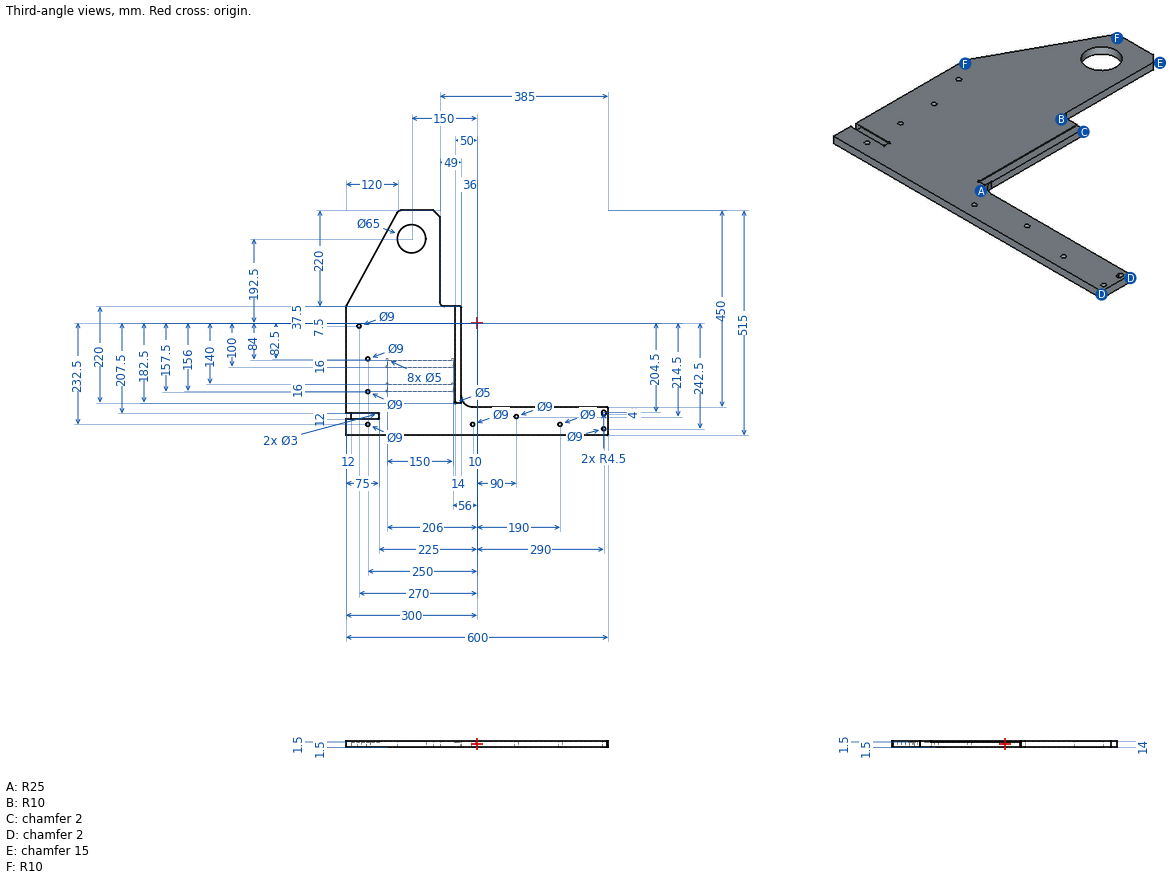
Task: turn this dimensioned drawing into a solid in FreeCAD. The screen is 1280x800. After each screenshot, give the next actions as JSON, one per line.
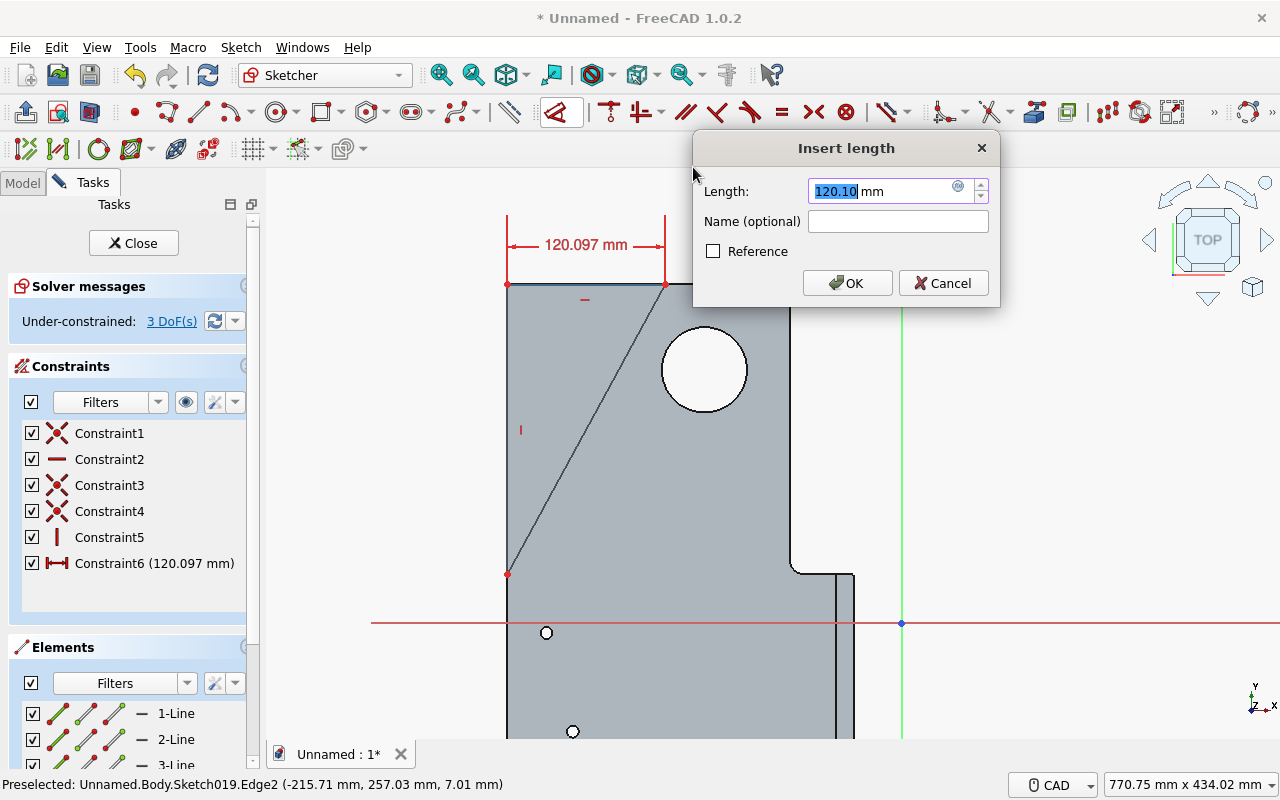
{"action": "type", "text": "120"}
{"action": "key", "text": "Return"}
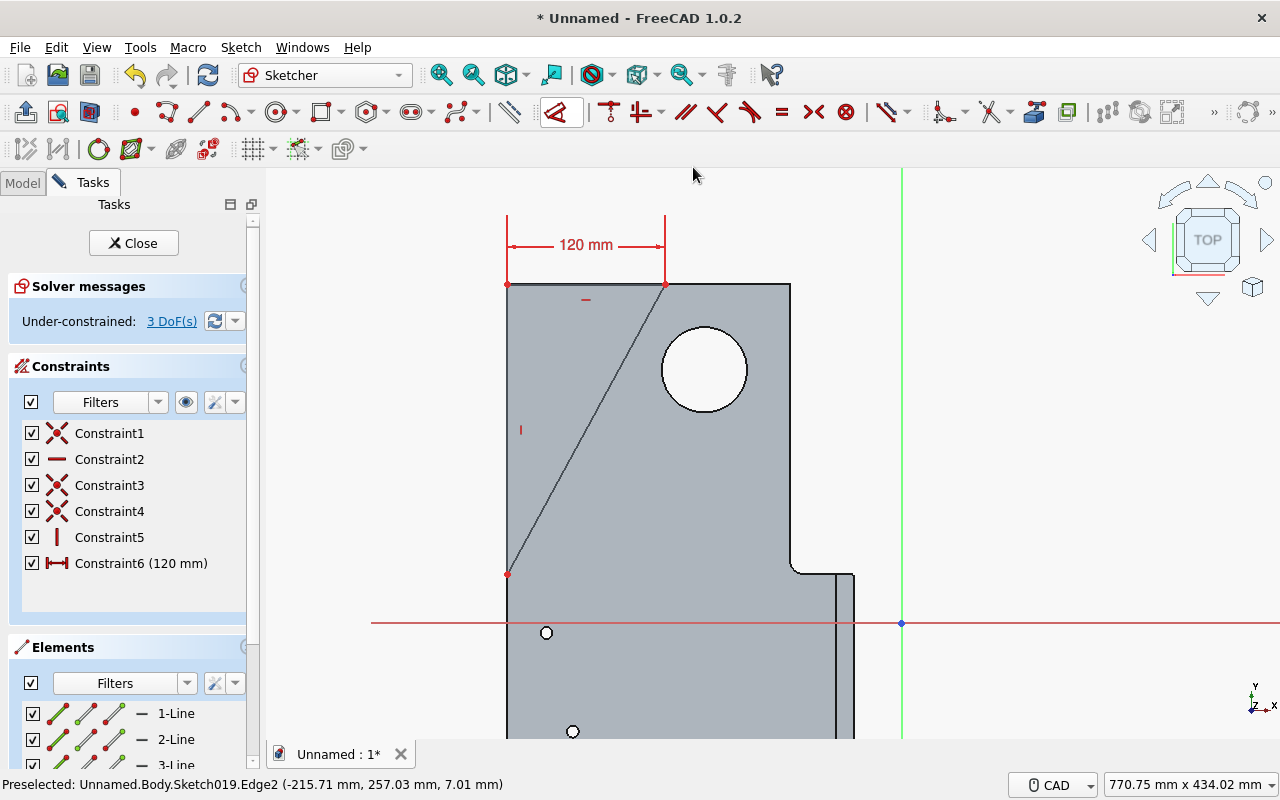
{"action": "left_click", "coordinate": [507, 372]}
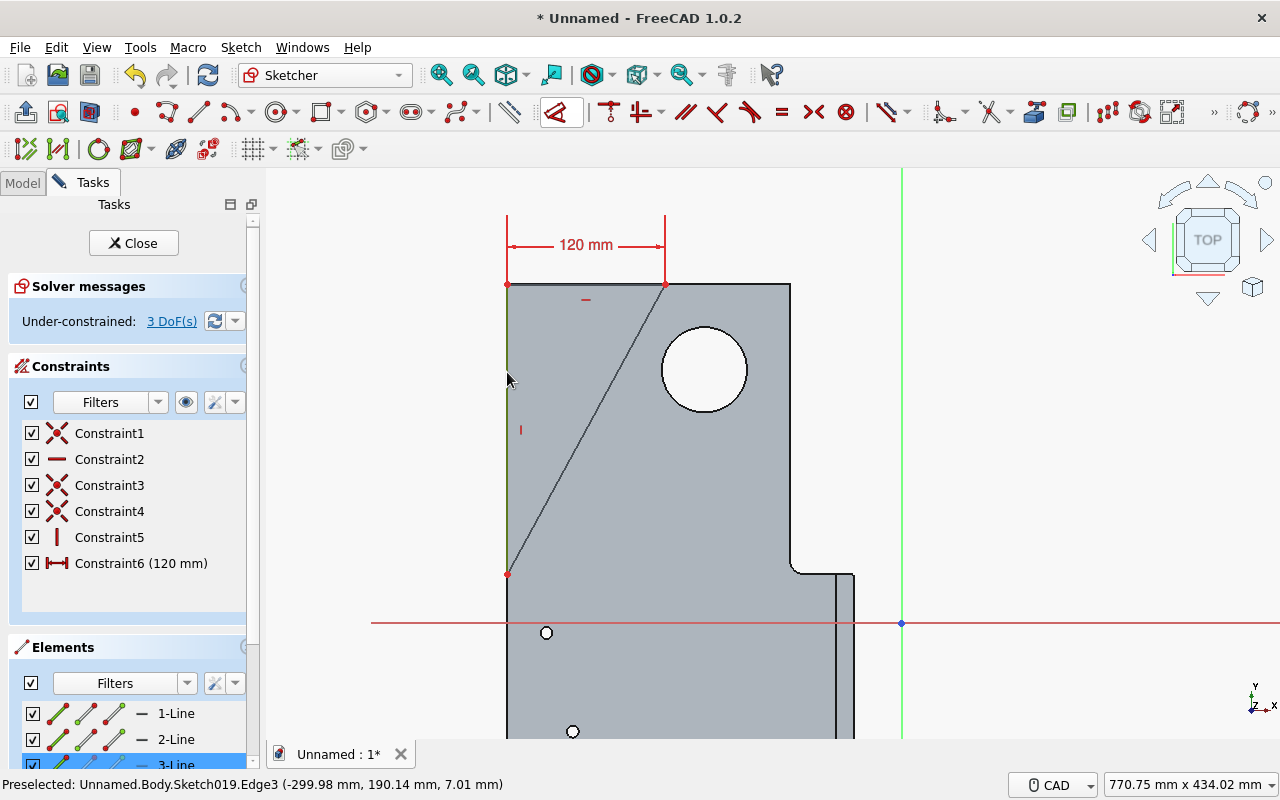
{"action": "left_click", "coordinate": [578, 112]}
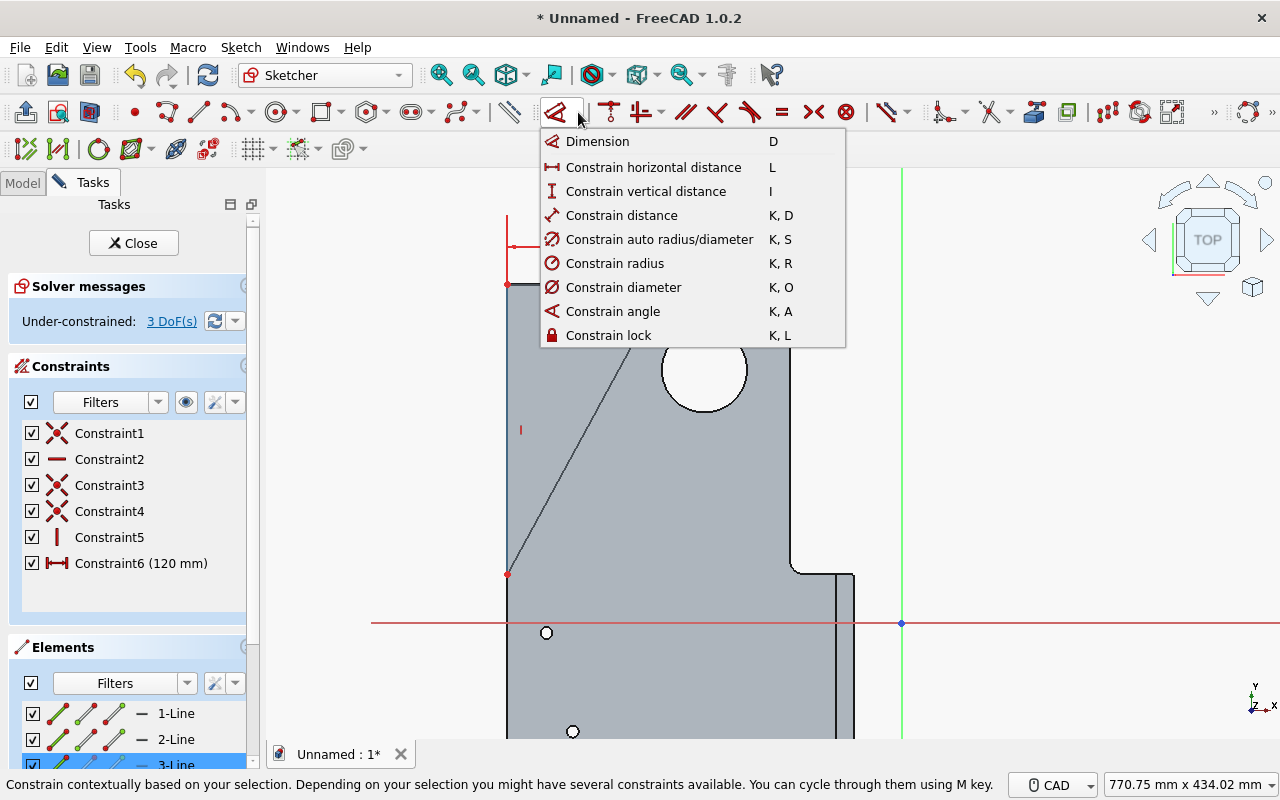
{"action": "left_click", "coordinate": [693, 191]}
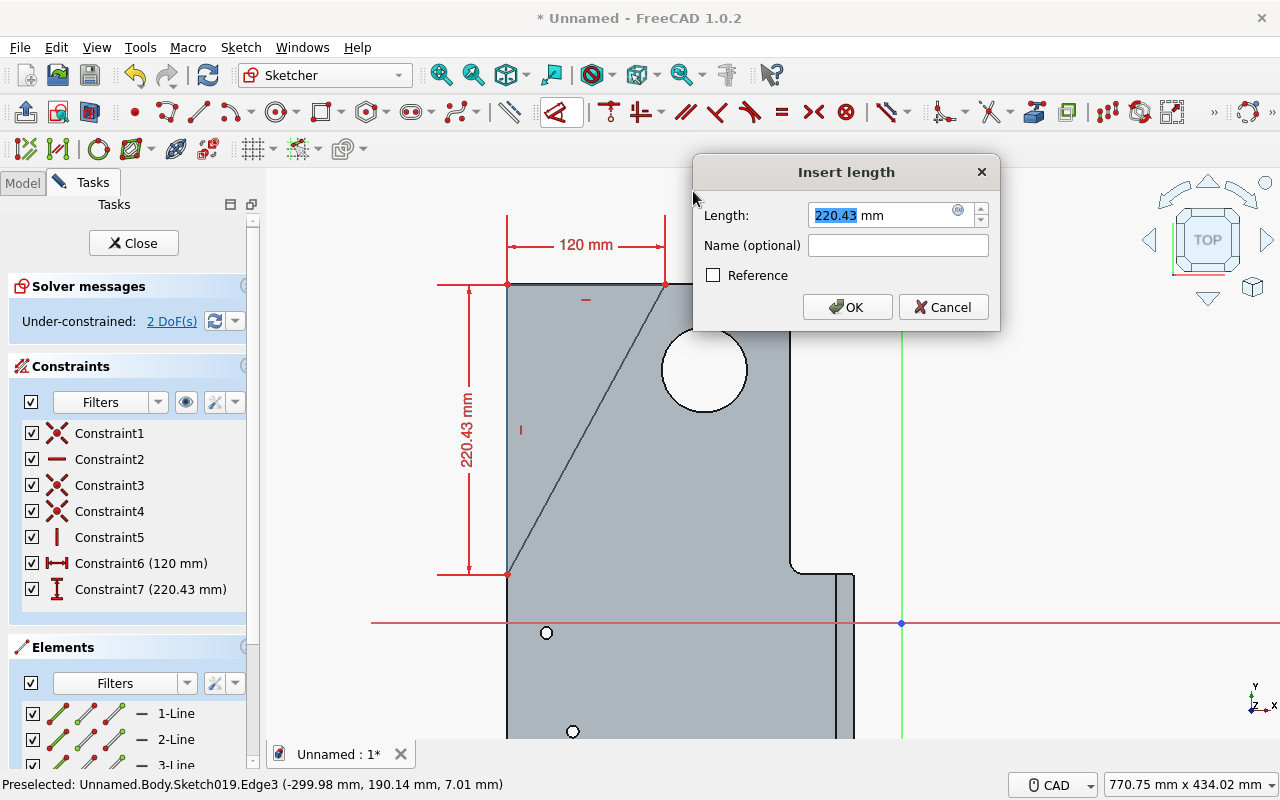
{"action": "type", "text": "220"}
{"action": "key", "text": "Return"}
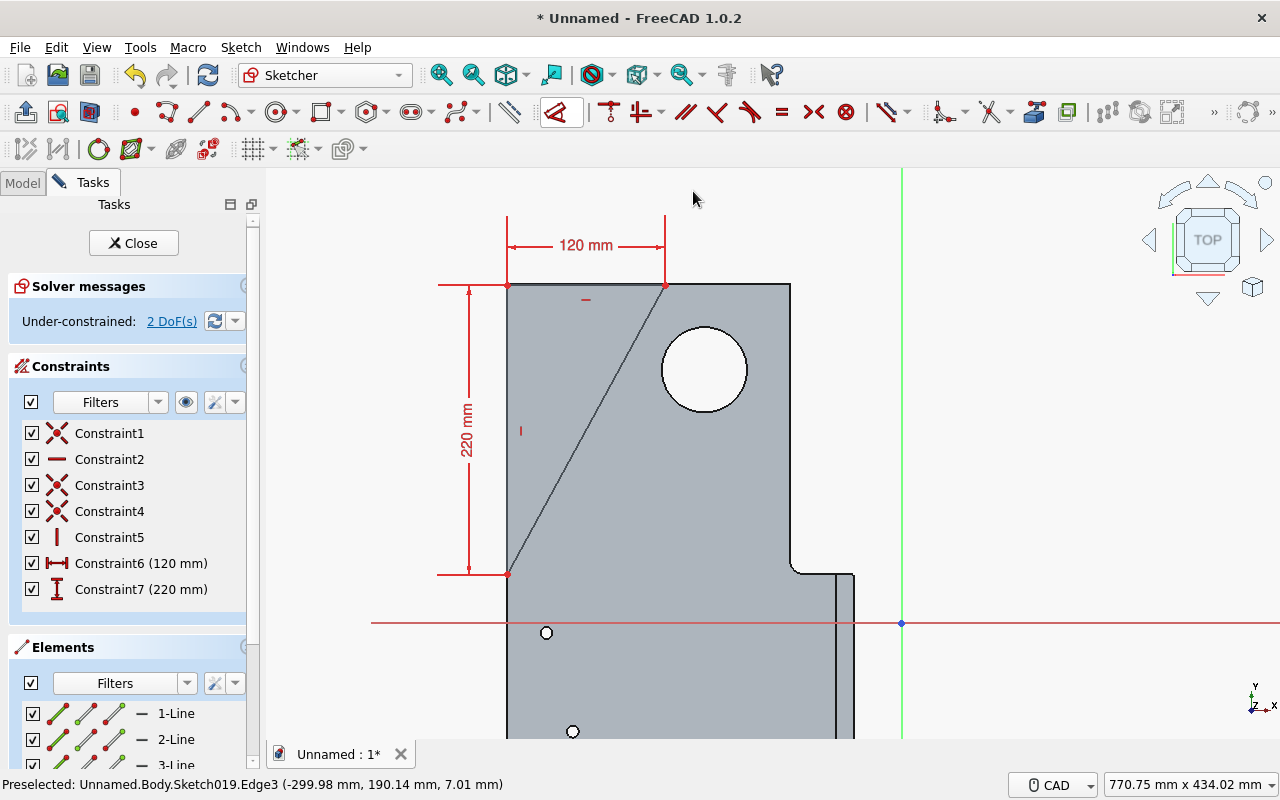
{"action": "left_click", "coordinate": [507, 575]}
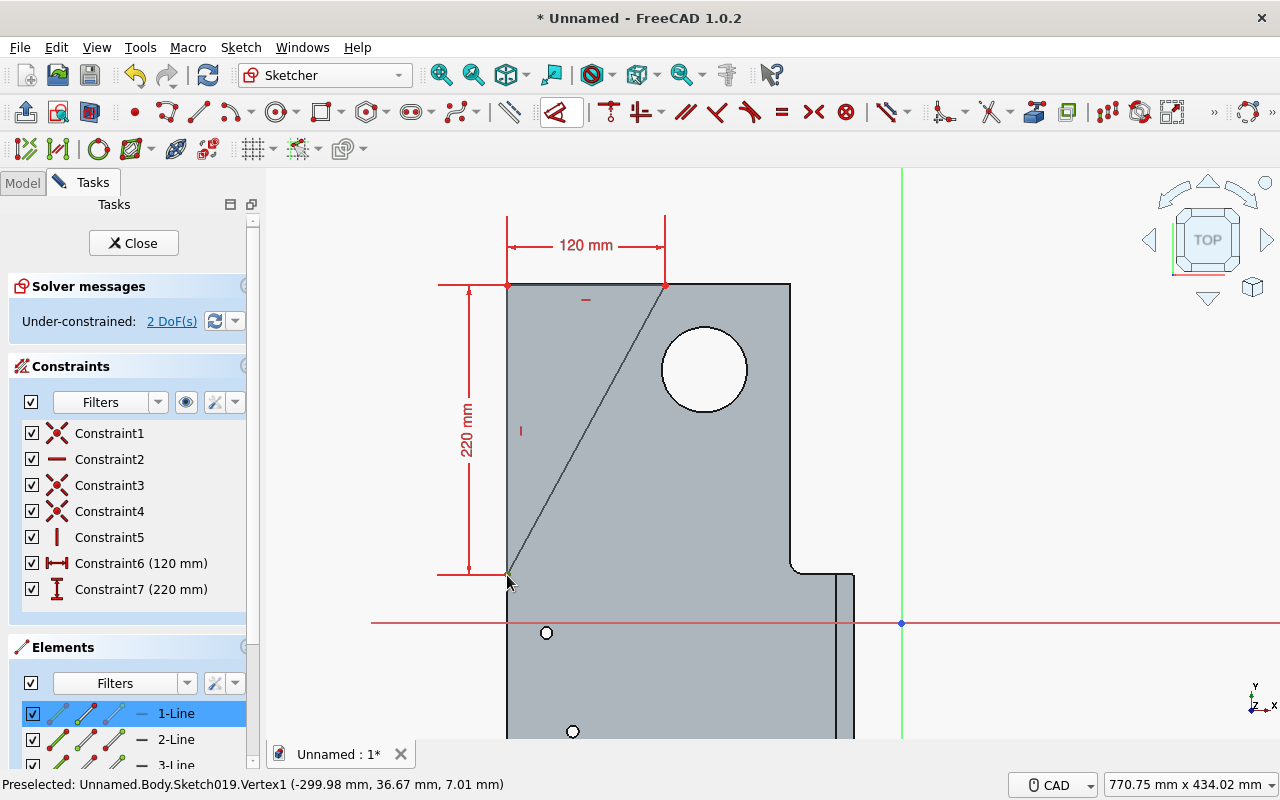
{"action": "key", "text": "l"}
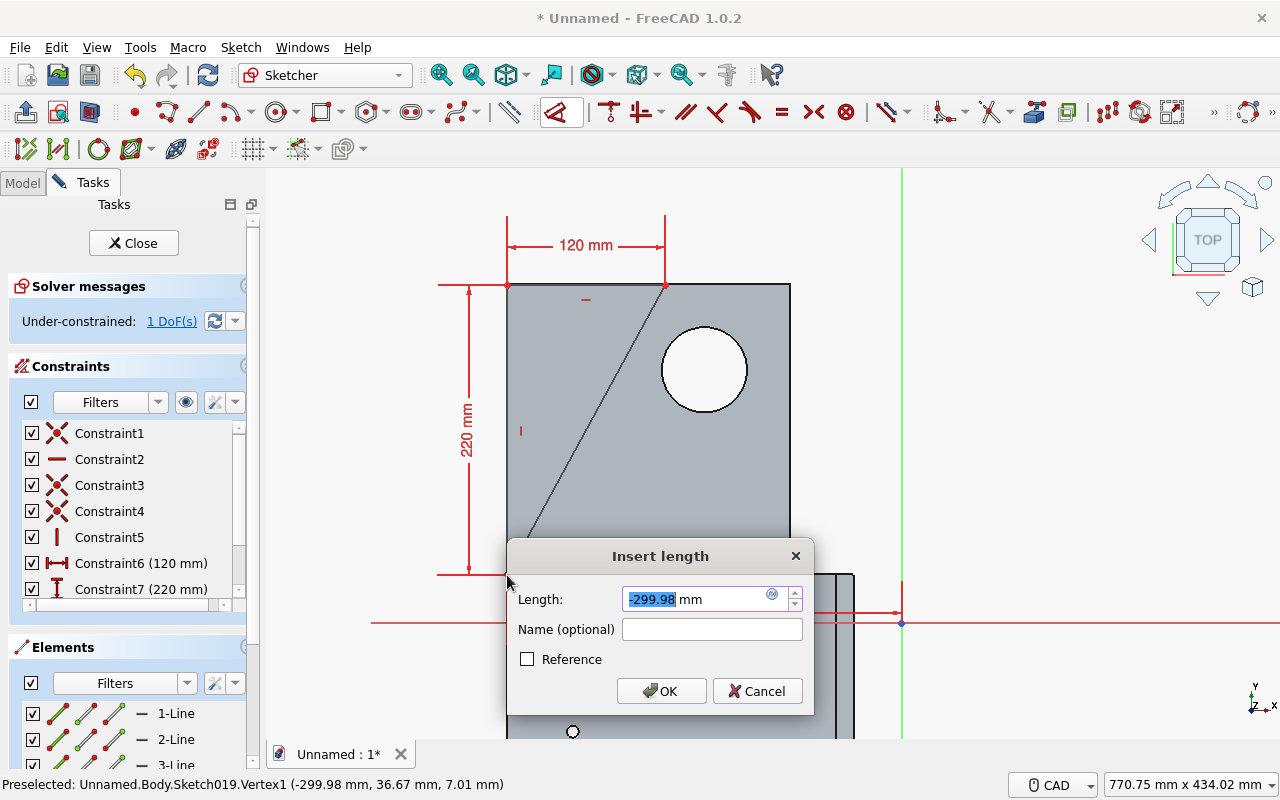
{"action": "type", "text": "-300"}
{"action": "key", "text": "Return"}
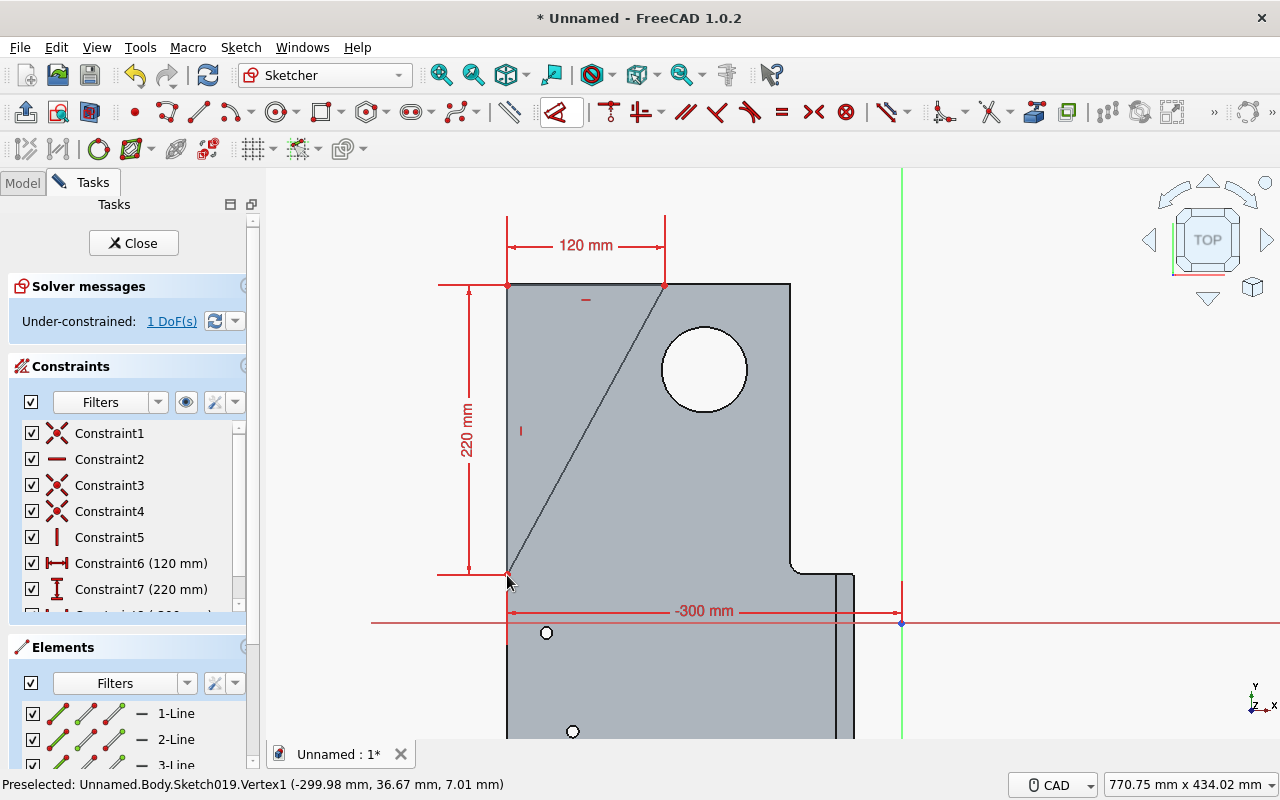
{"action": "left_click", "coordinate": [507, 575]}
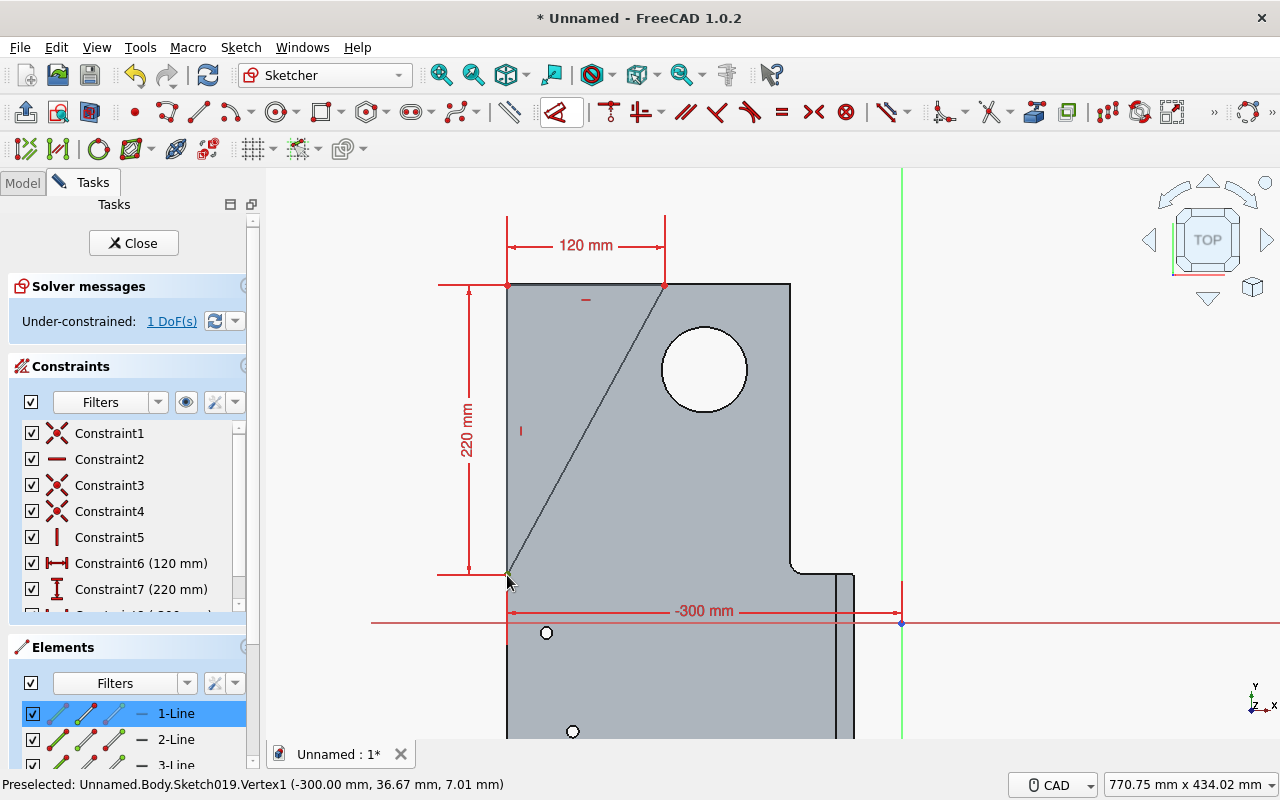
{"action": "key", "text": "i"}